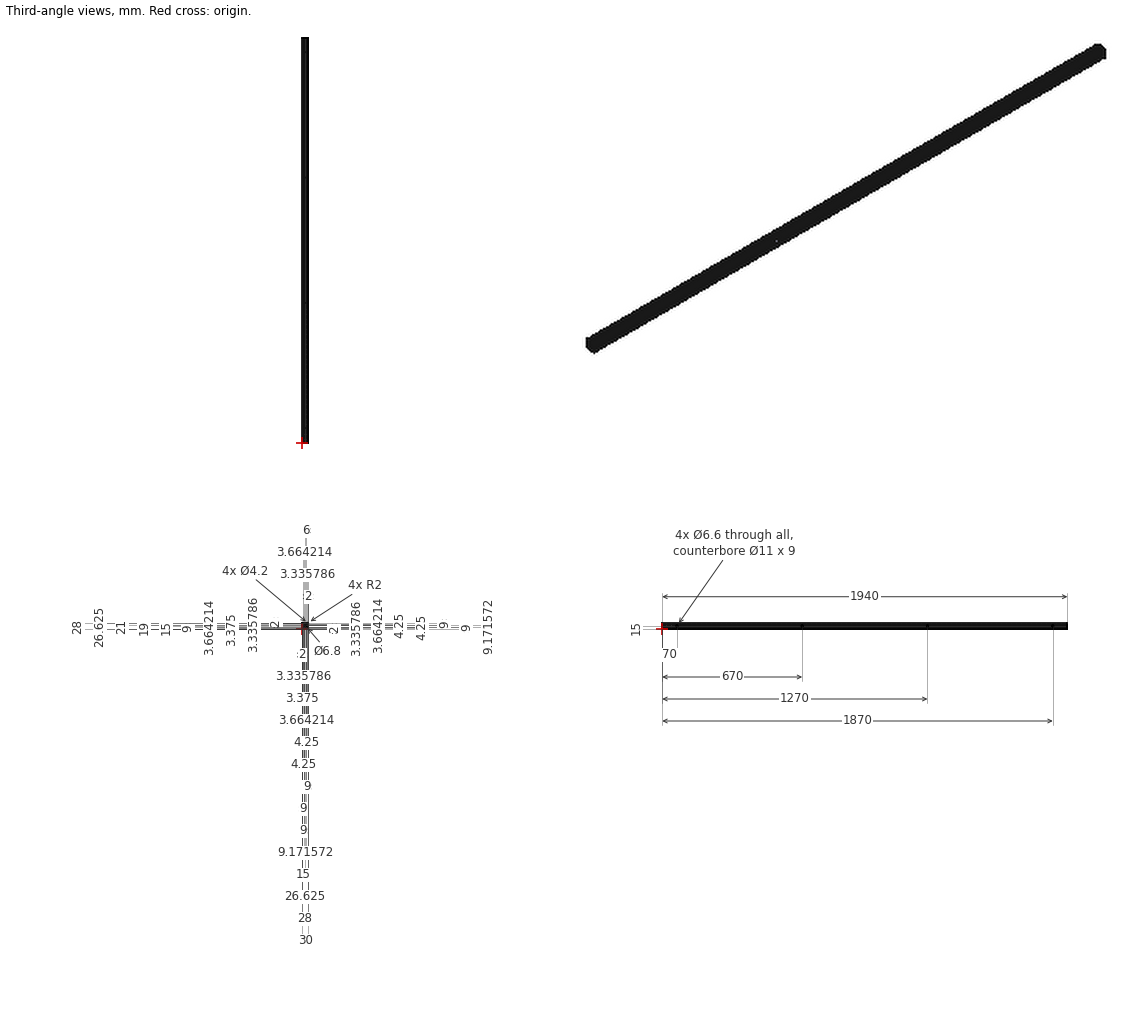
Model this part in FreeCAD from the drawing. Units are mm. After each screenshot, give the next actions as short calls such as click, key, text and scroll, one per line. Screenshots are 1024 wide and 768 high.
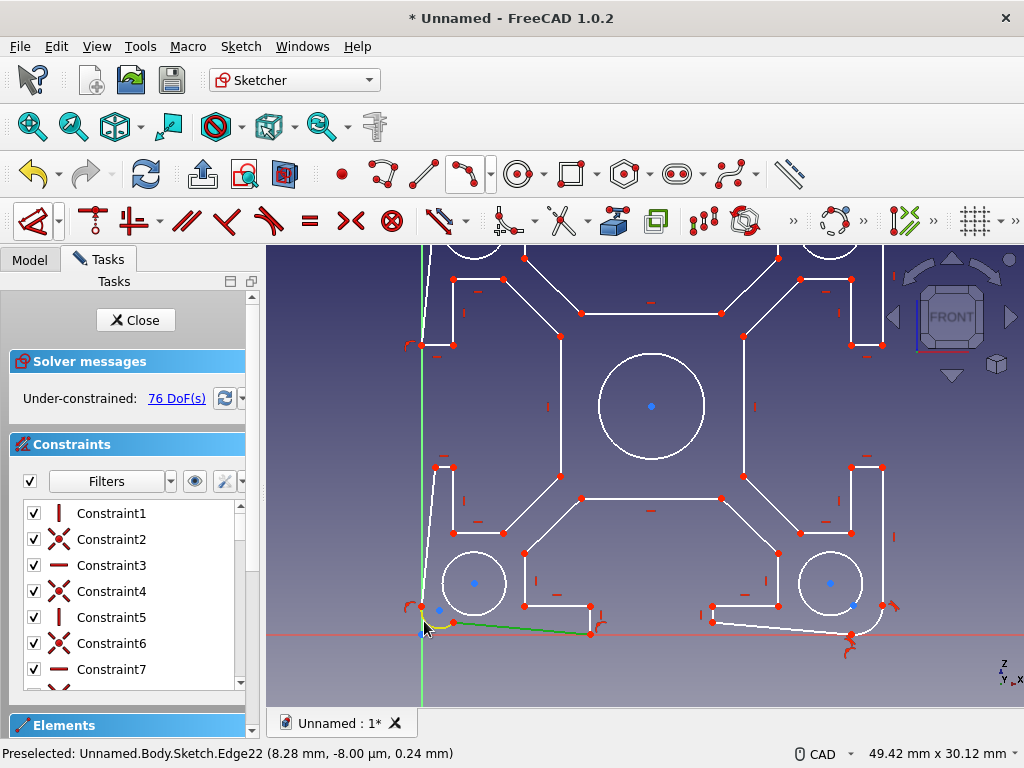
click(424, 620)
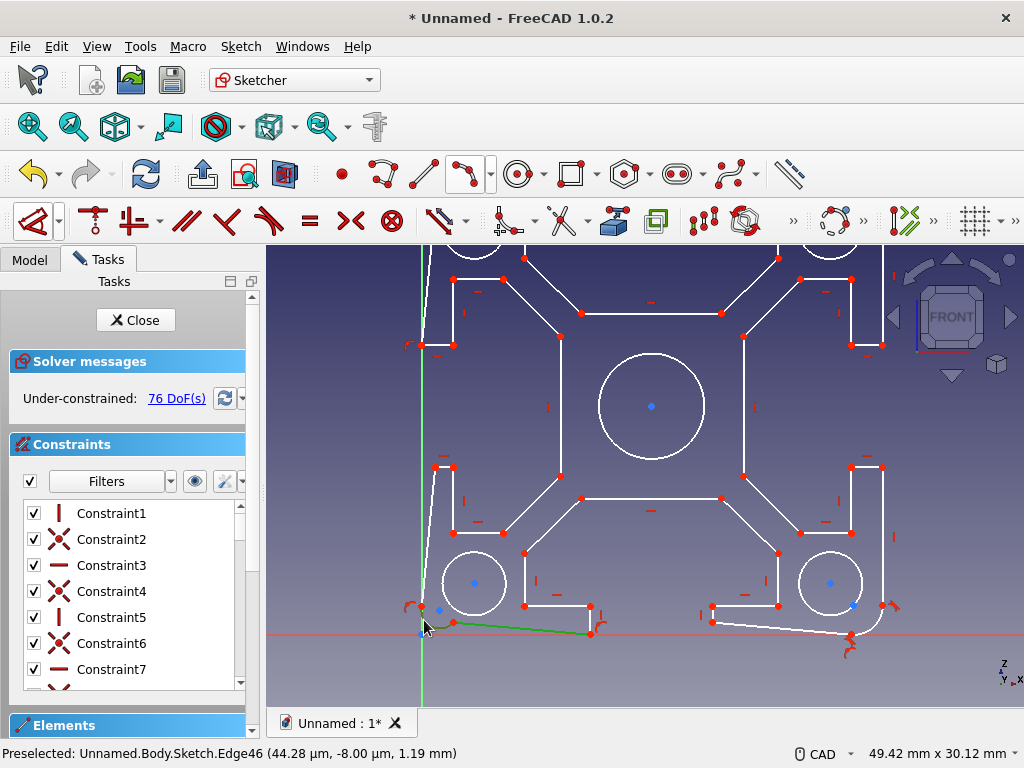
click(269, 222)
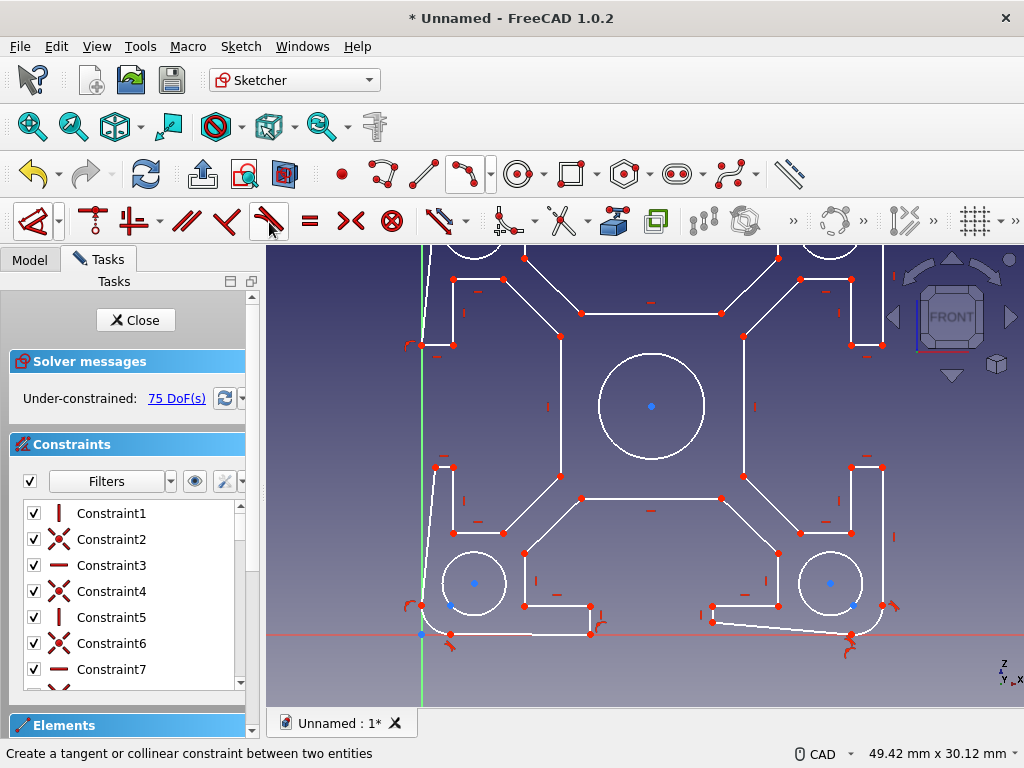
scroll(431, 509, up, 2)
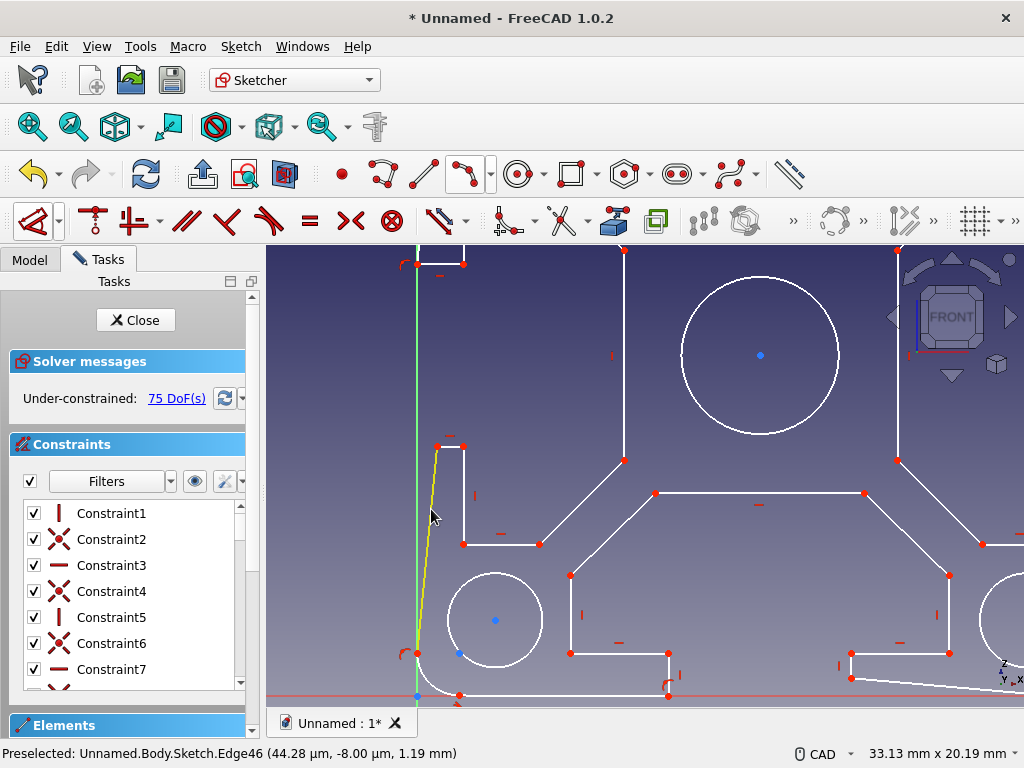
click(431, 509)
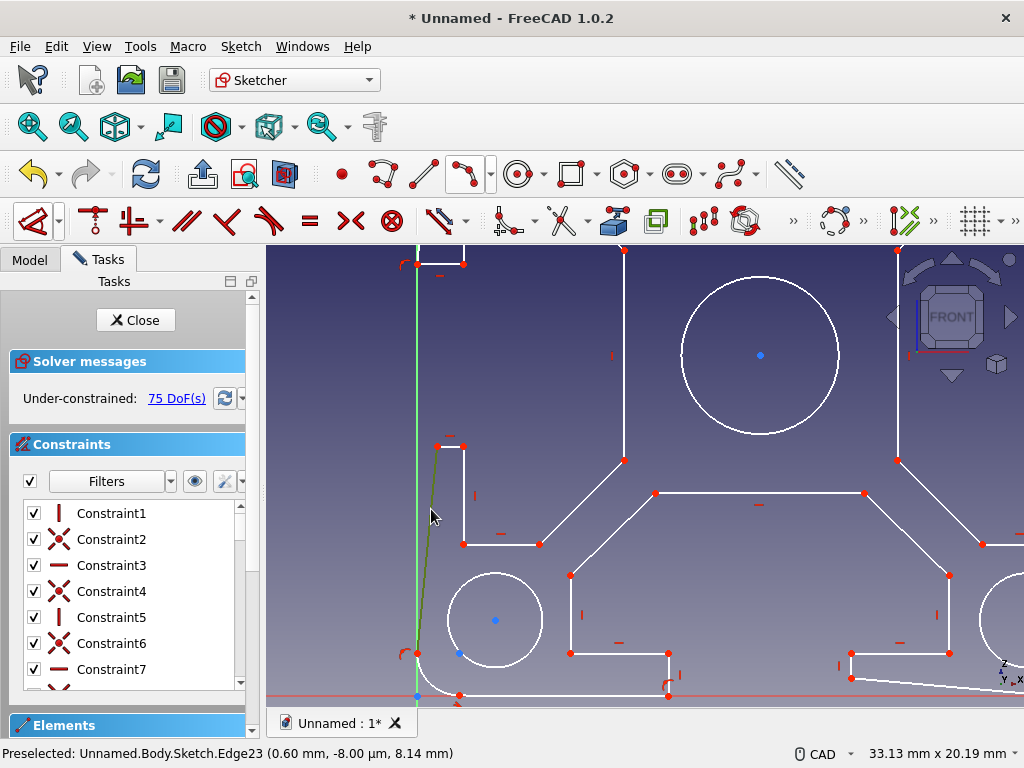
click(419, 666)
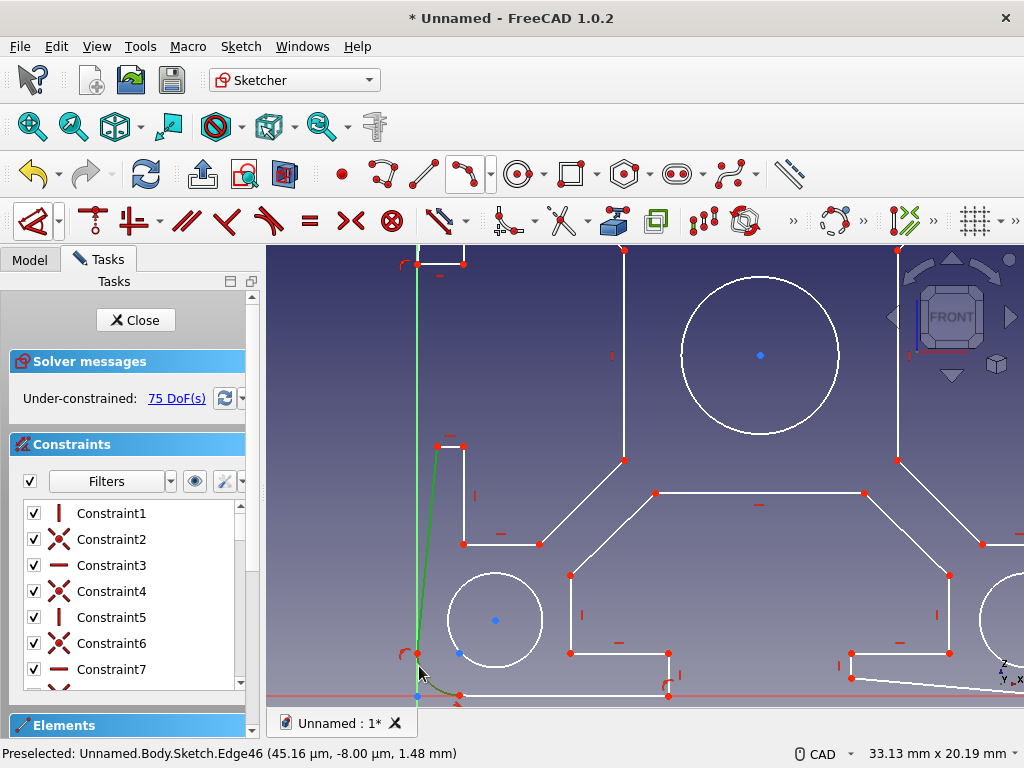
click(269, 222)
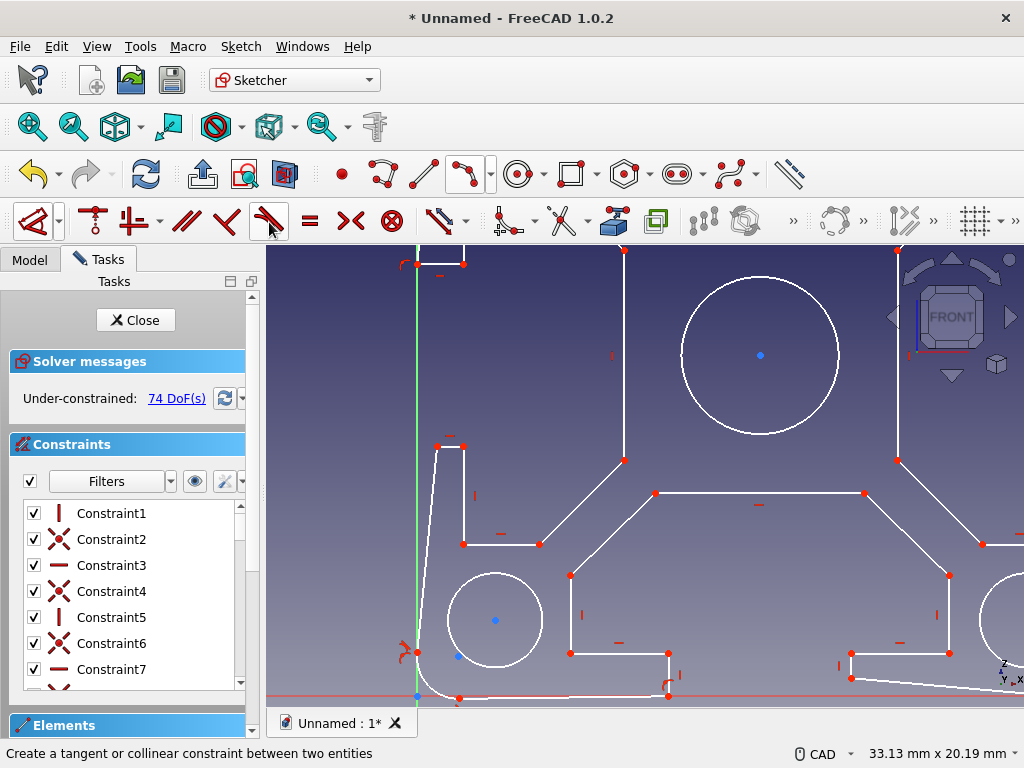
scroll(426, 576, down, 4)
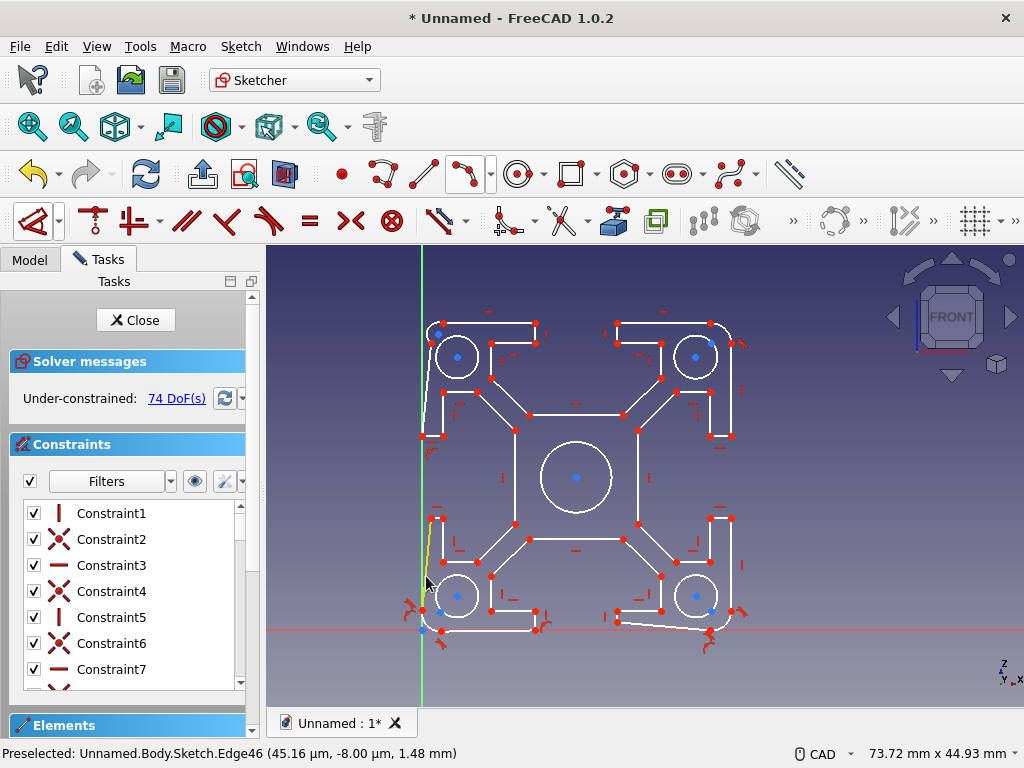
scroll(428, 371, up, 4)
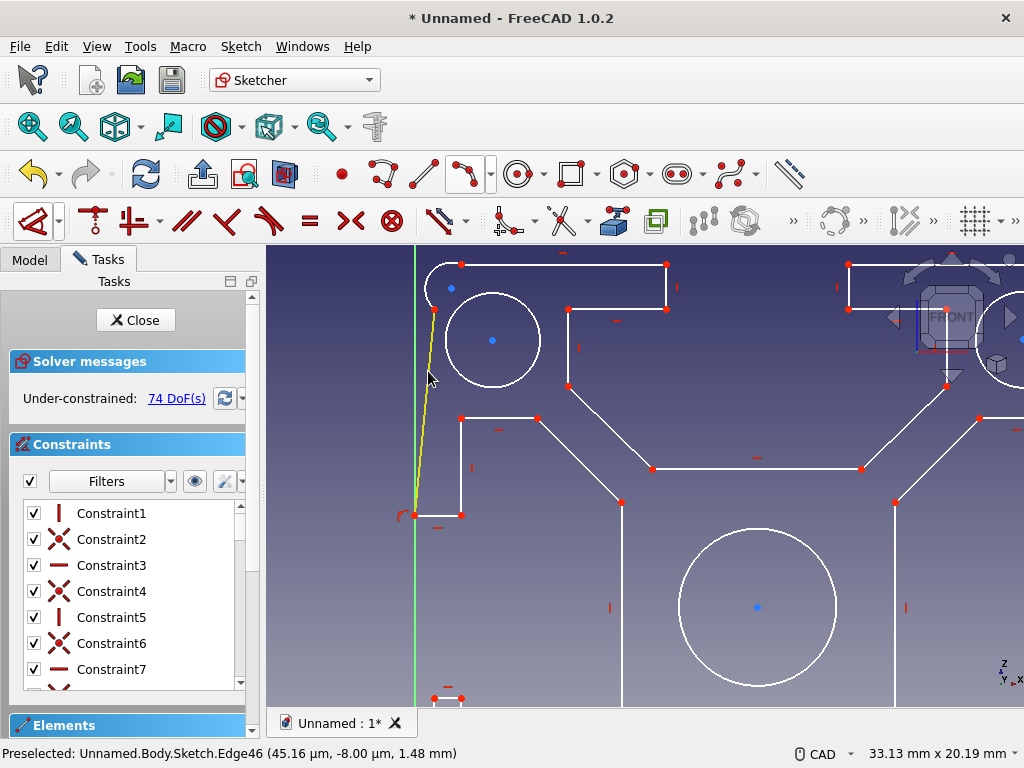
click(429, 371)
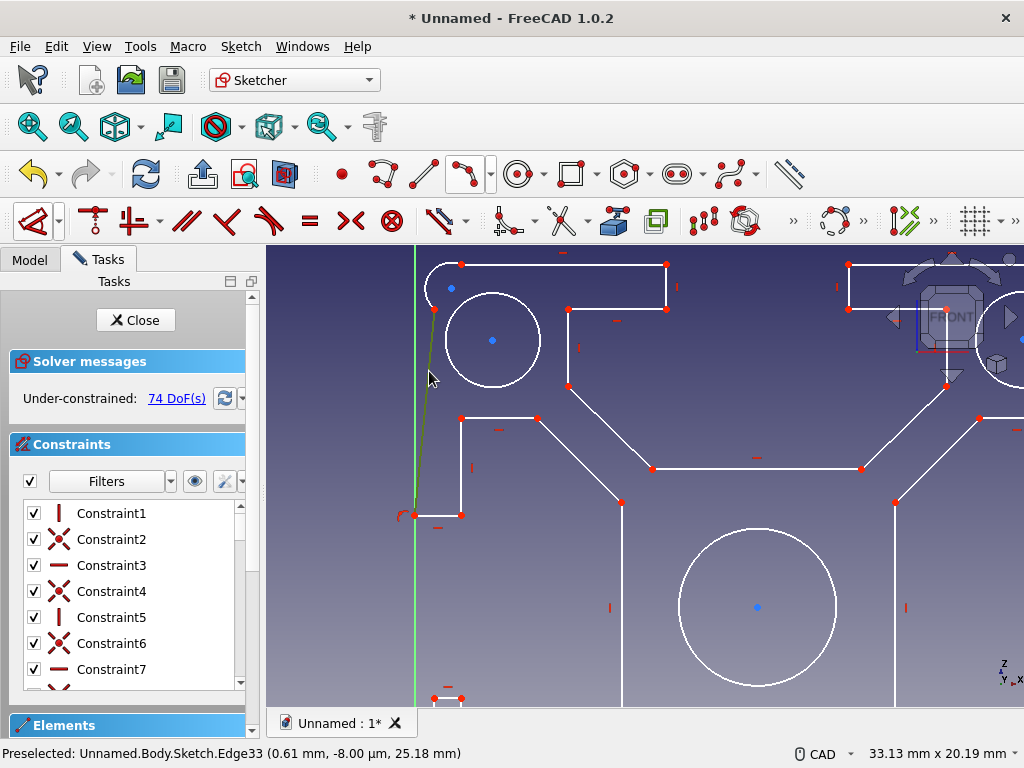
scroll(425, 290, up, 2)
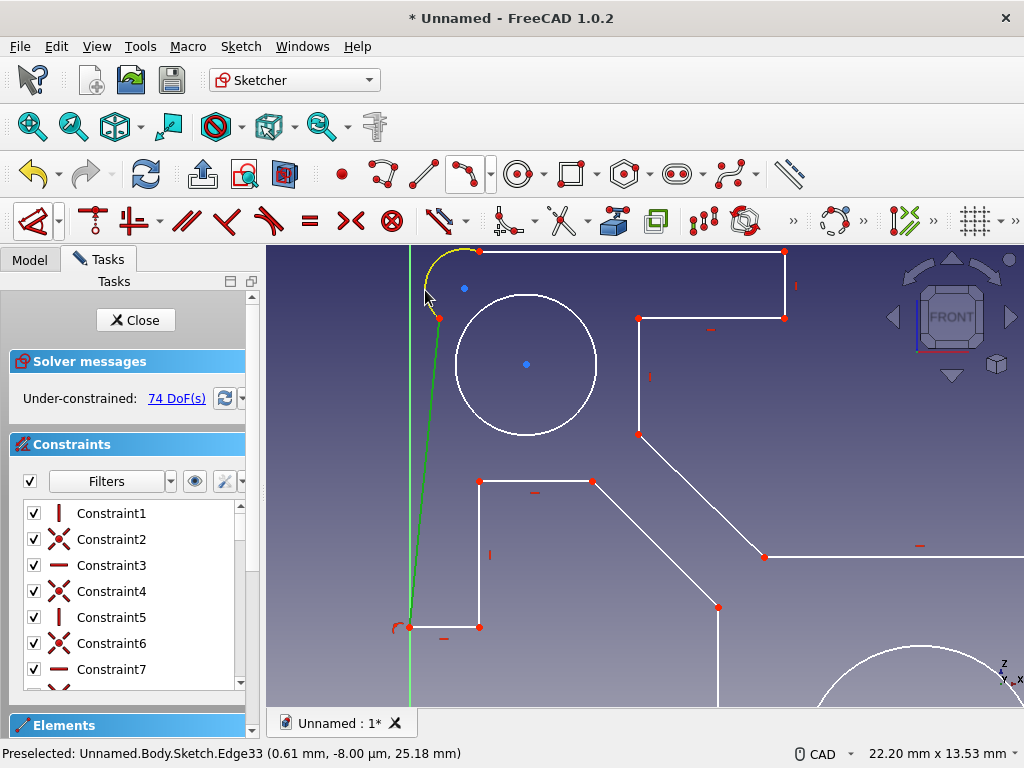
click(425, 289)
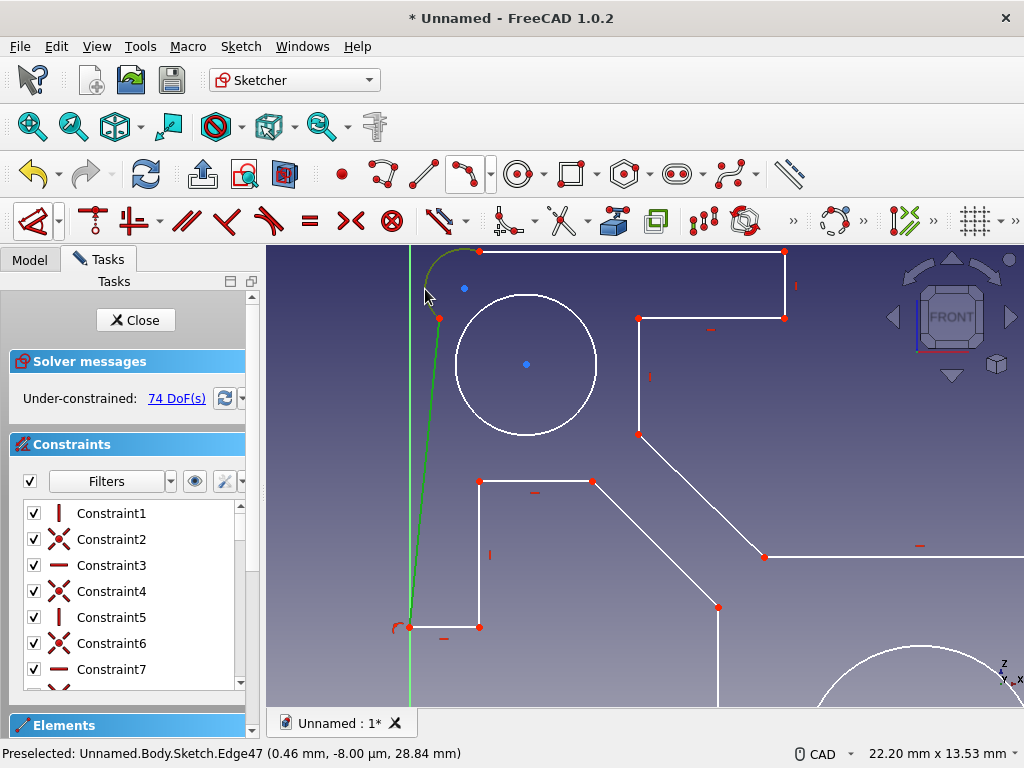
click(269, 222)